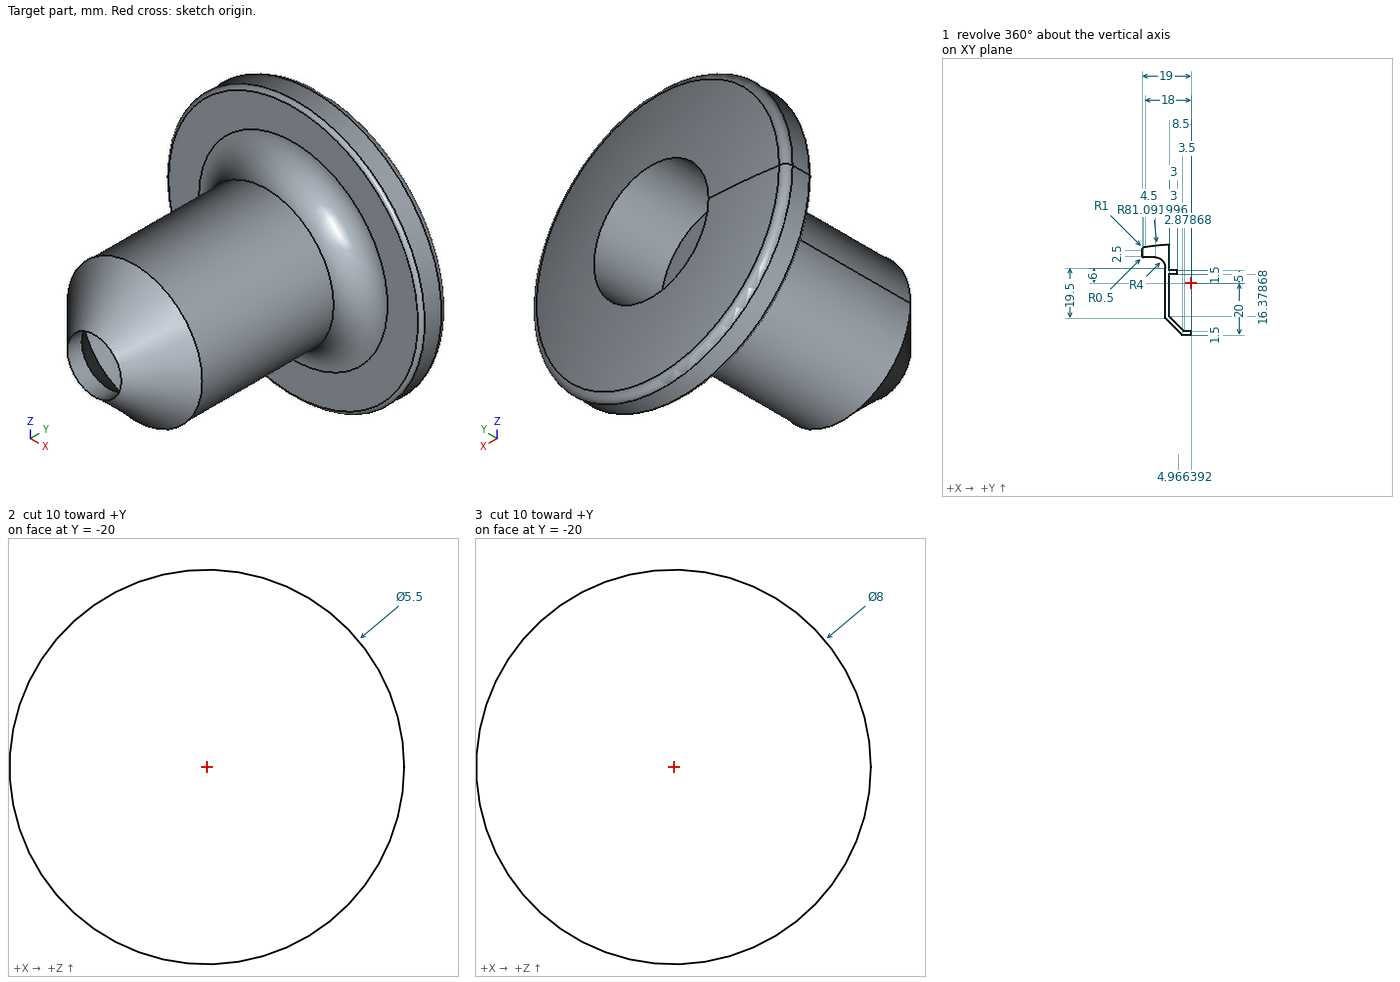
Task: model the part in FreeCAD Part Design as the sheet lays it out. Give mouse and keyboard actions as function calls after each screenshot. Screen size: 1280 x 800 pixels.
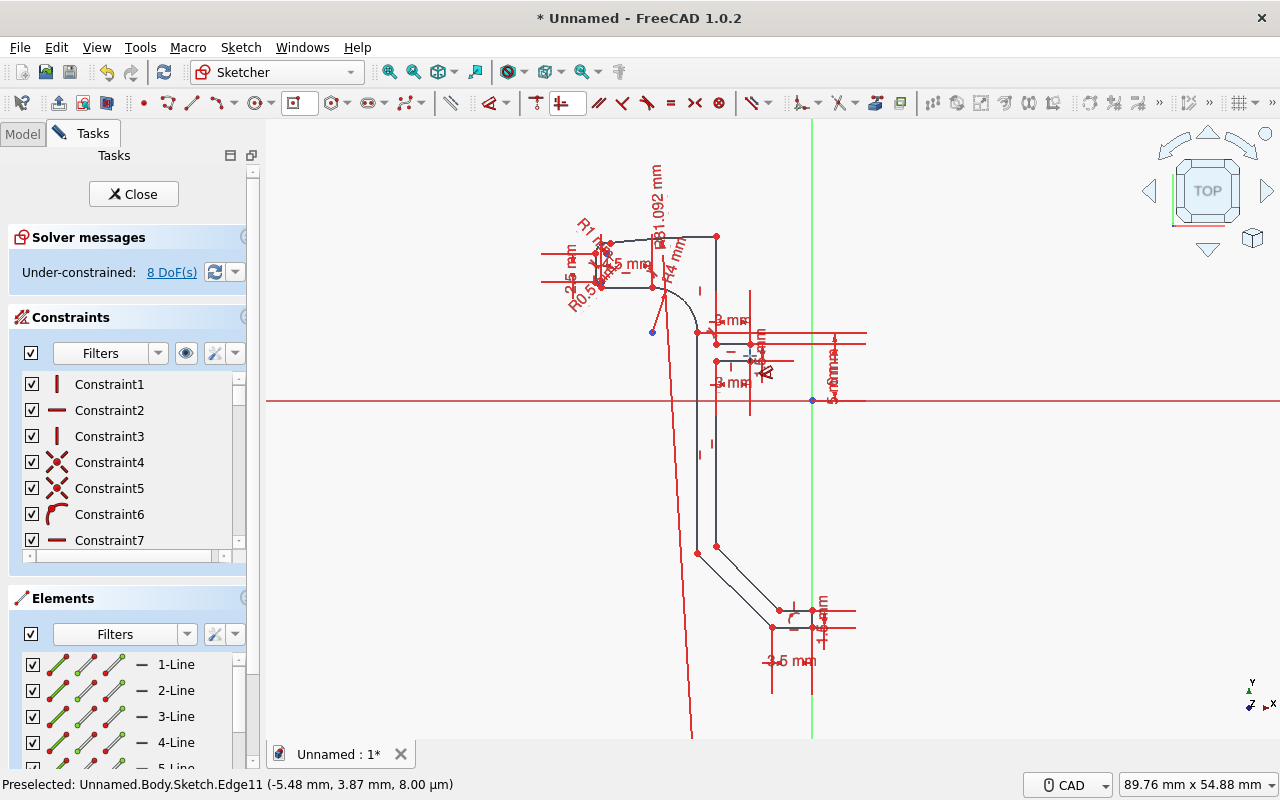
click(596, 254)
click(754, 220)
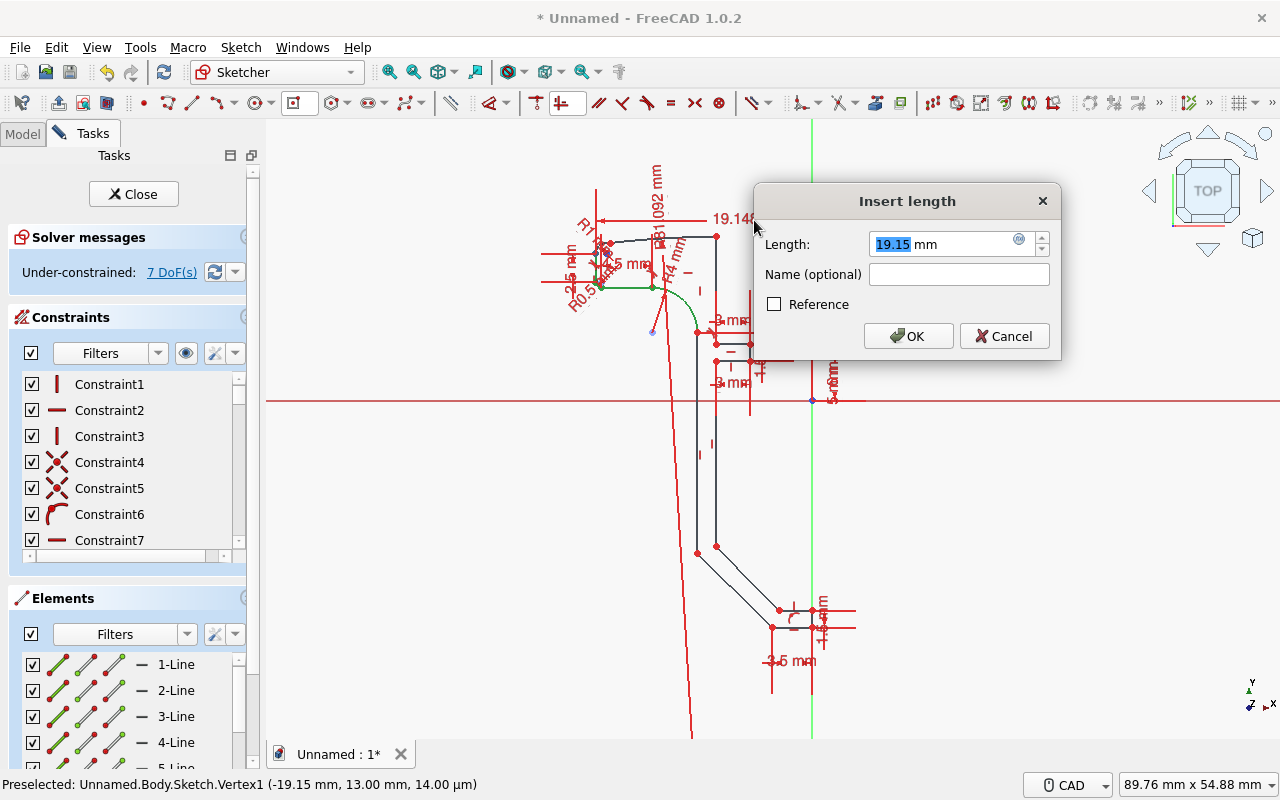
text(19)
key(Return)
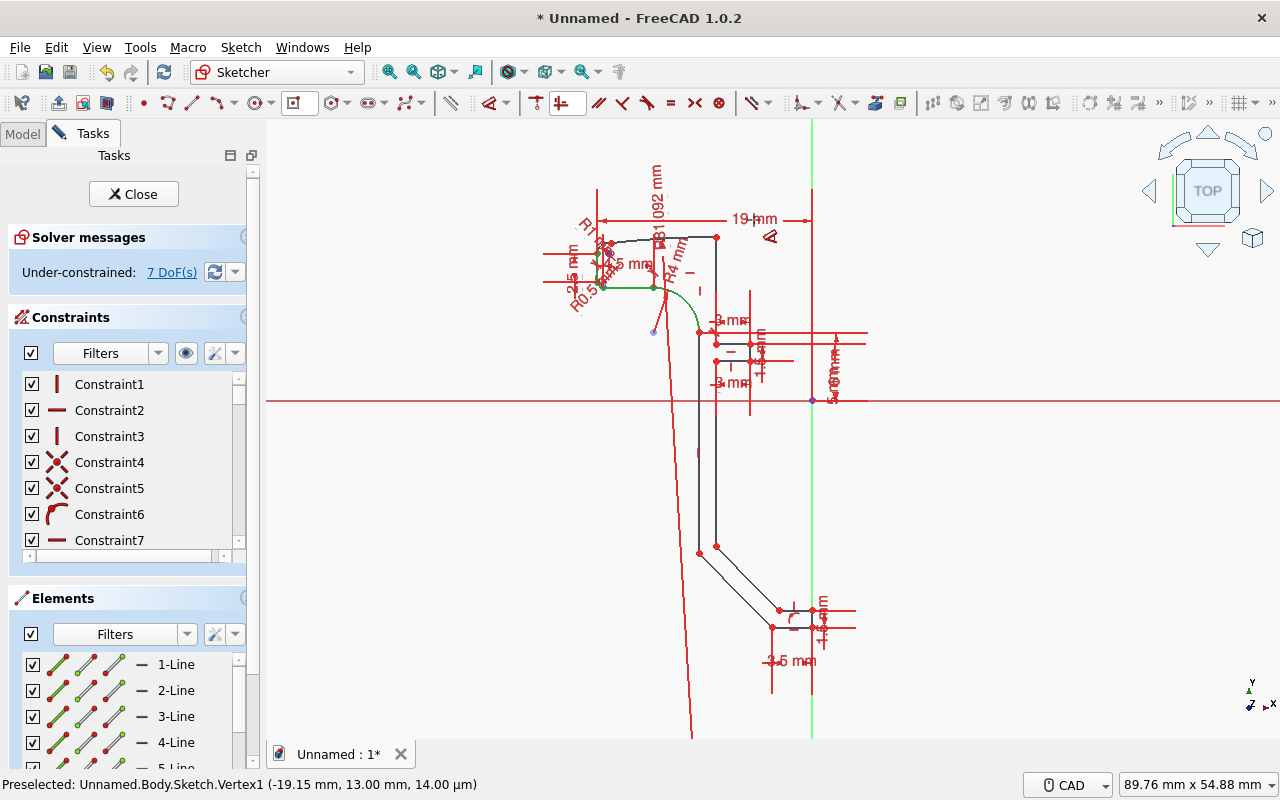
click(772, 628)
click(846, 514)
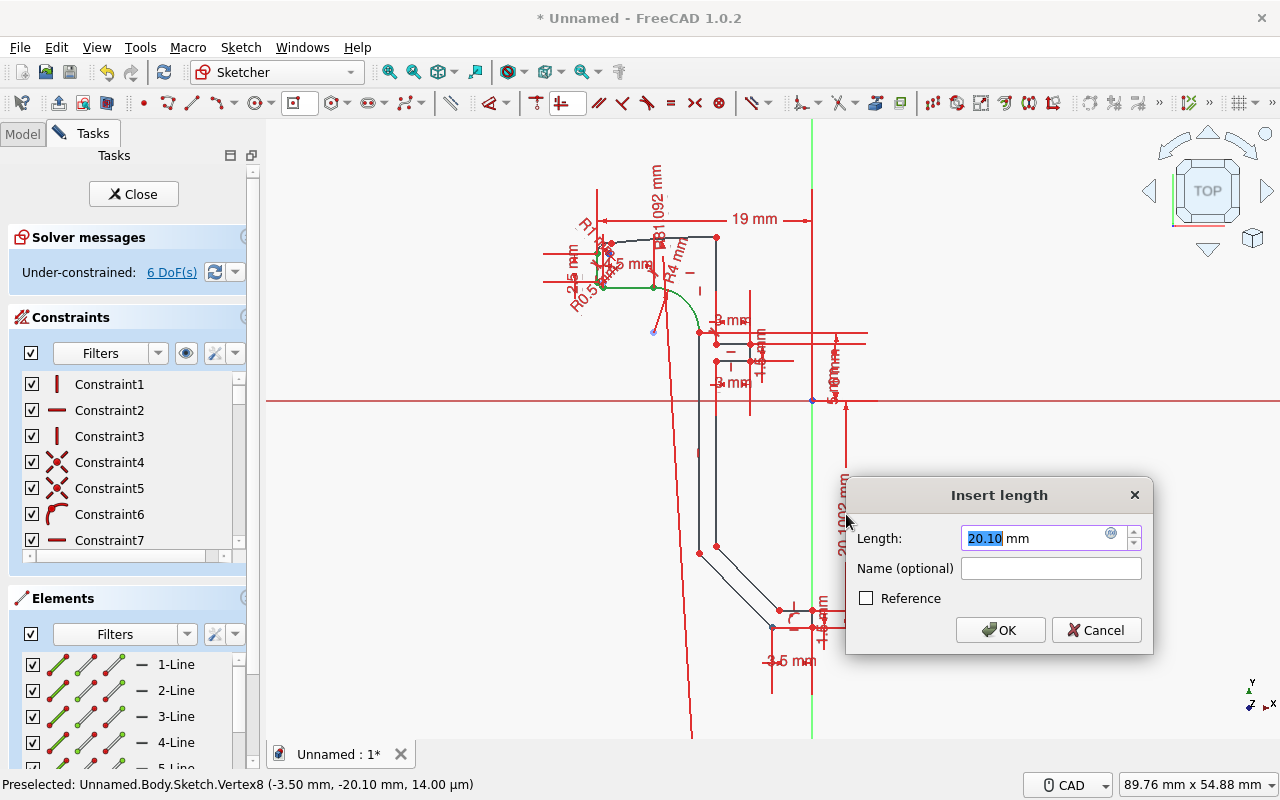
text(20)
key(Return)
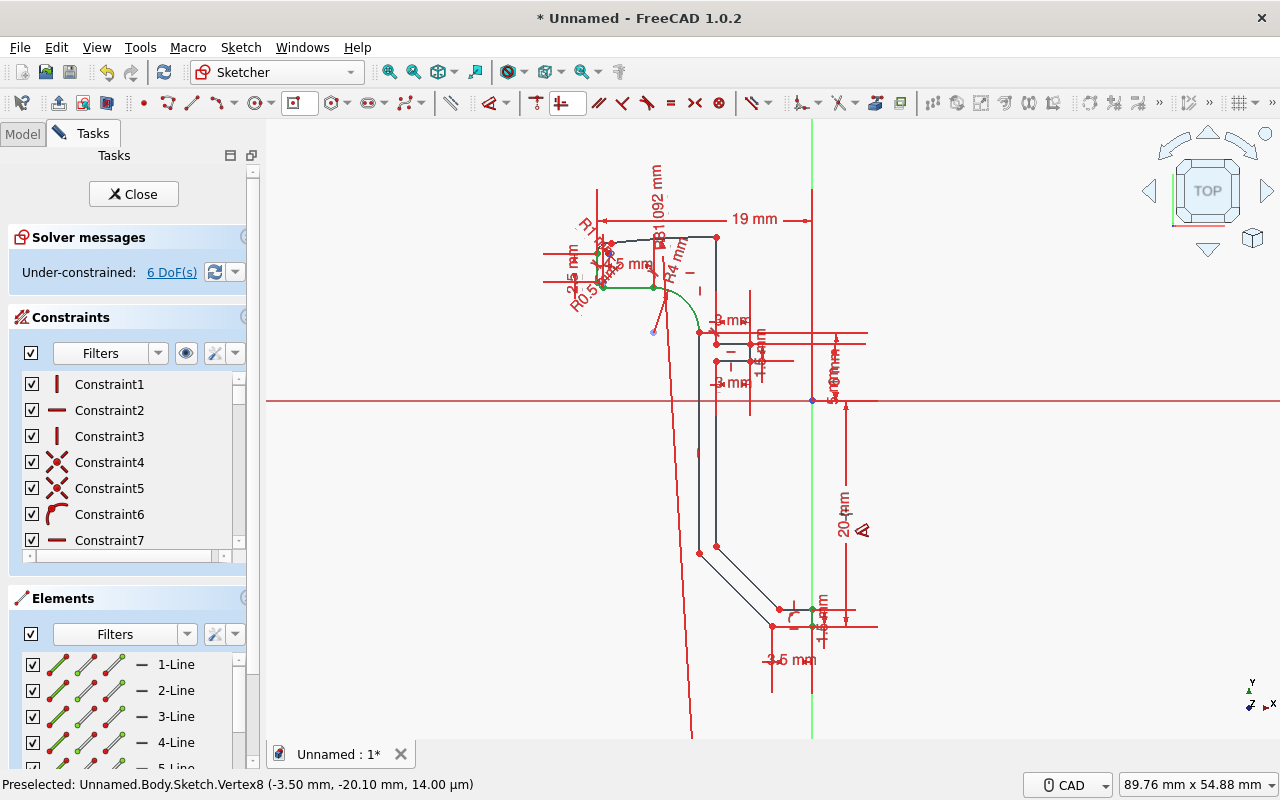
click(612, 243)
click(666, 435)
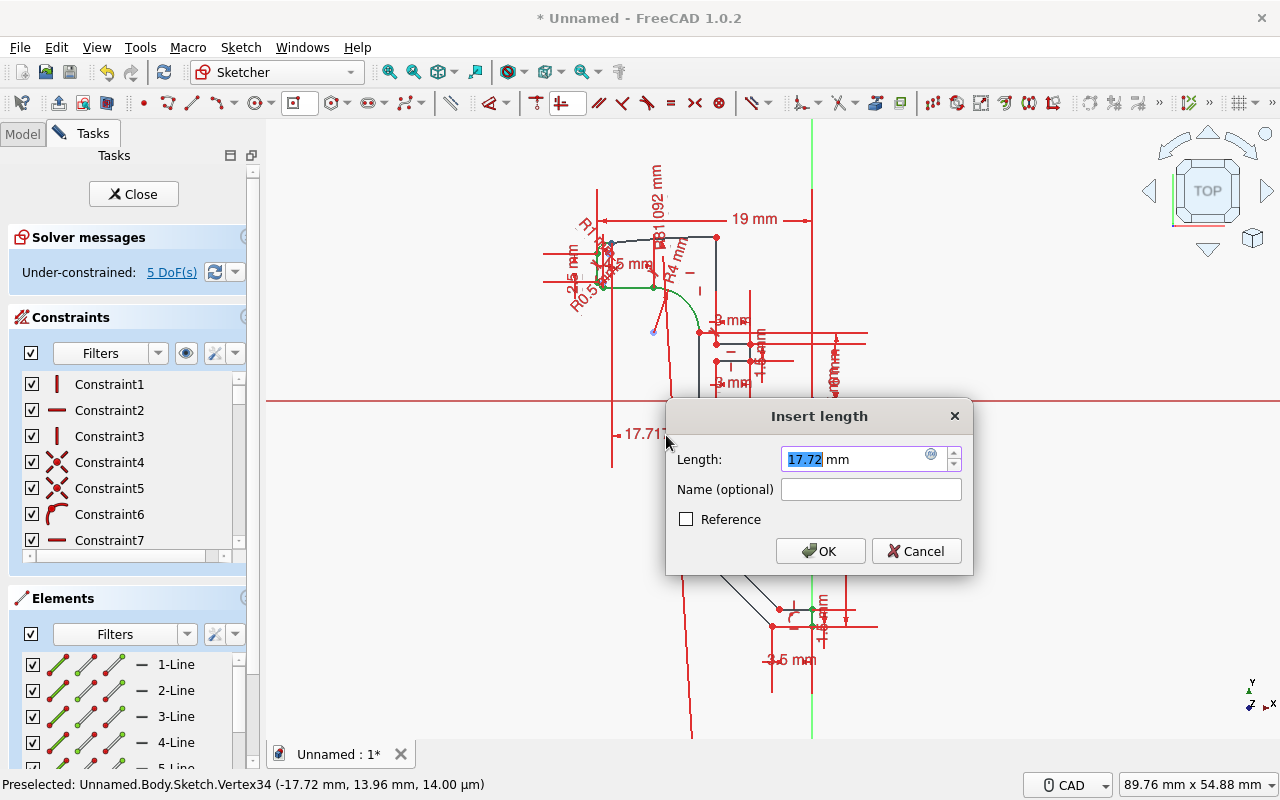
text(18)
key(Return)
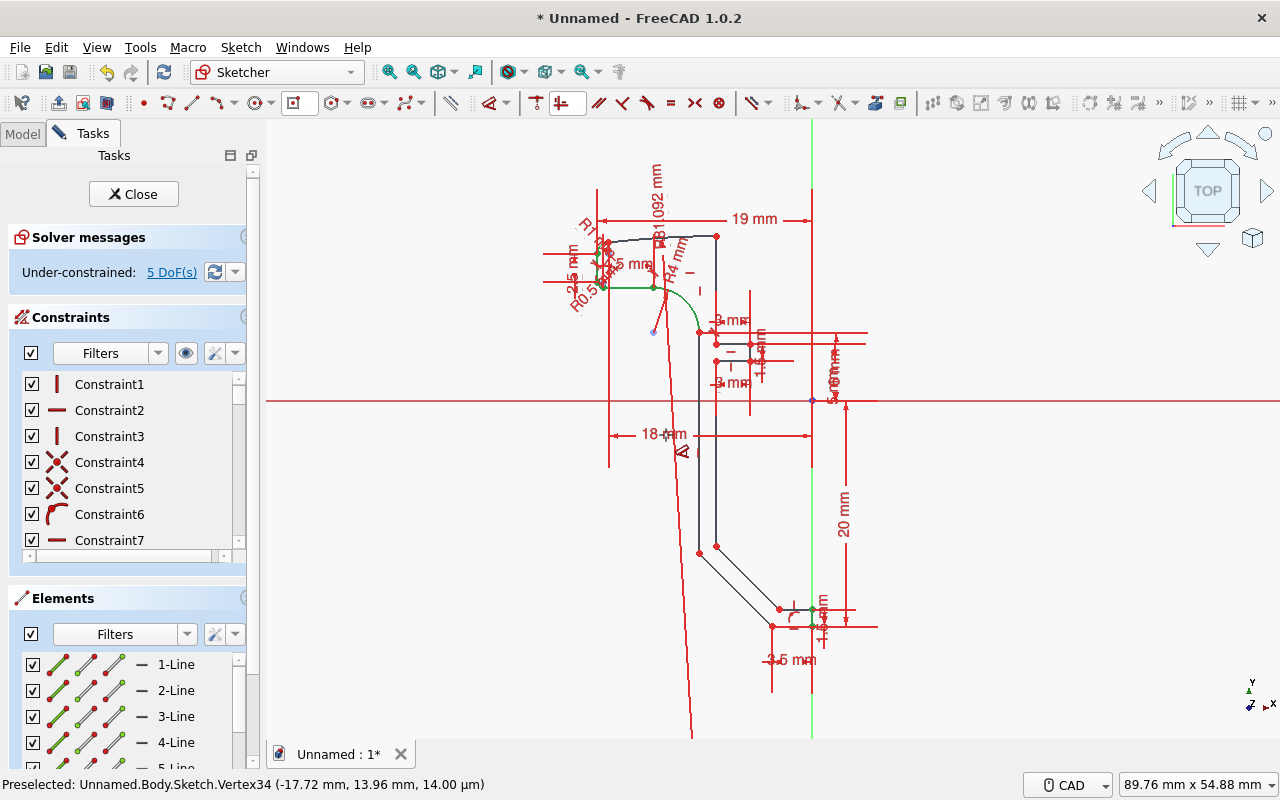
click(699, 399)
click(665, 494)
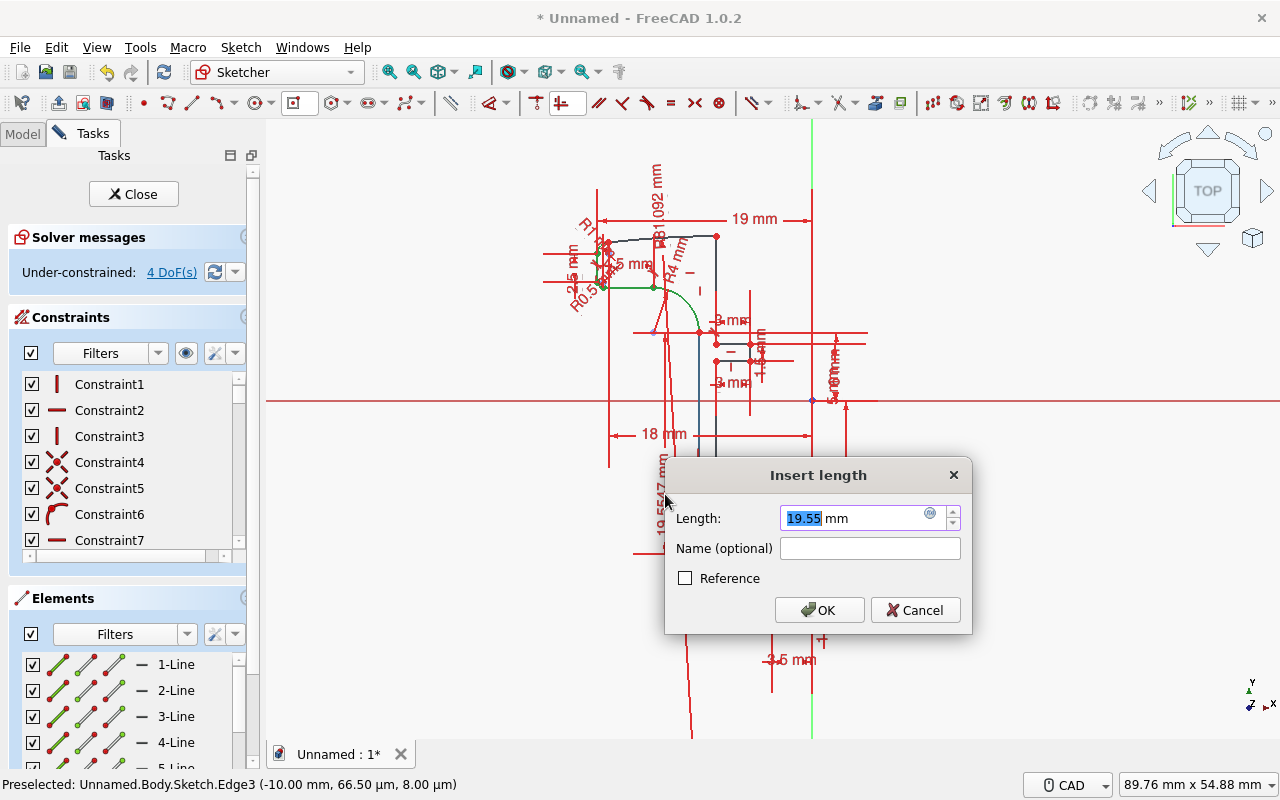
text(19.5)
key(Return)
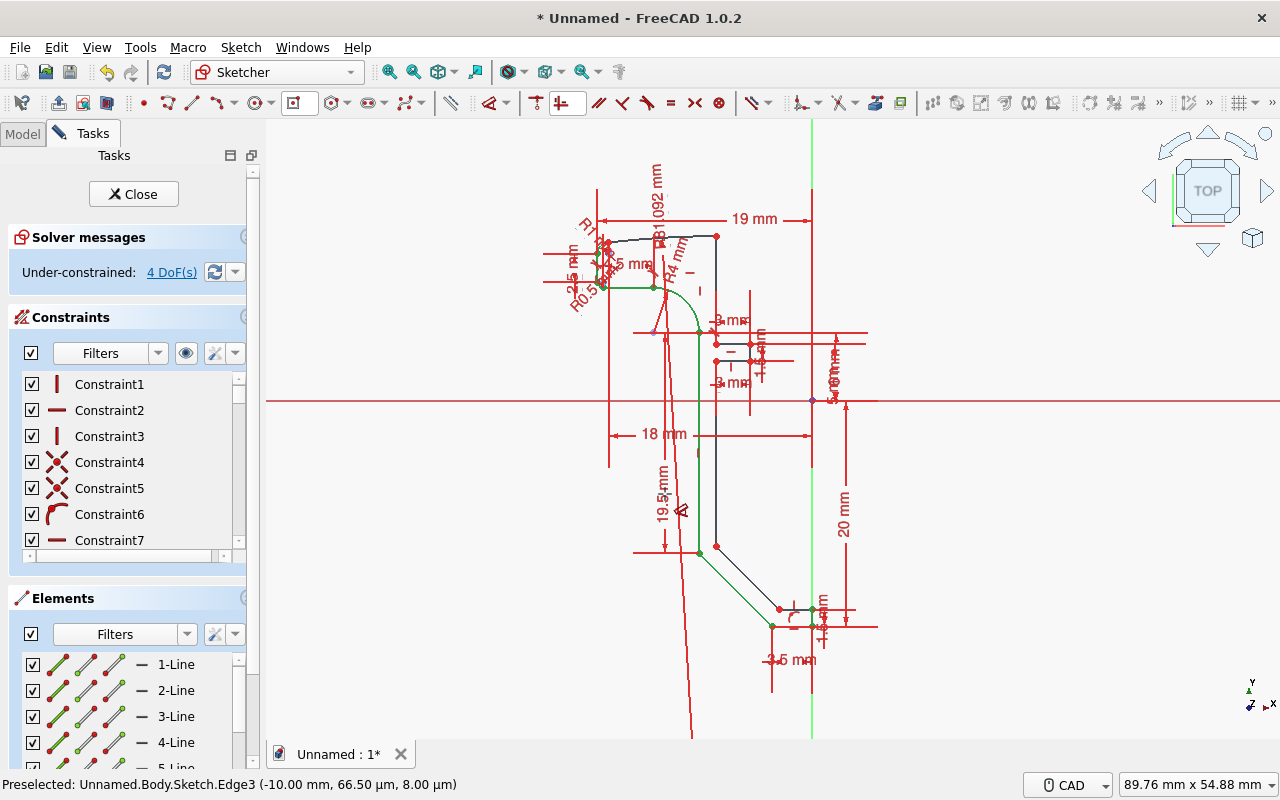
click(716, 547)
click(786, 581)